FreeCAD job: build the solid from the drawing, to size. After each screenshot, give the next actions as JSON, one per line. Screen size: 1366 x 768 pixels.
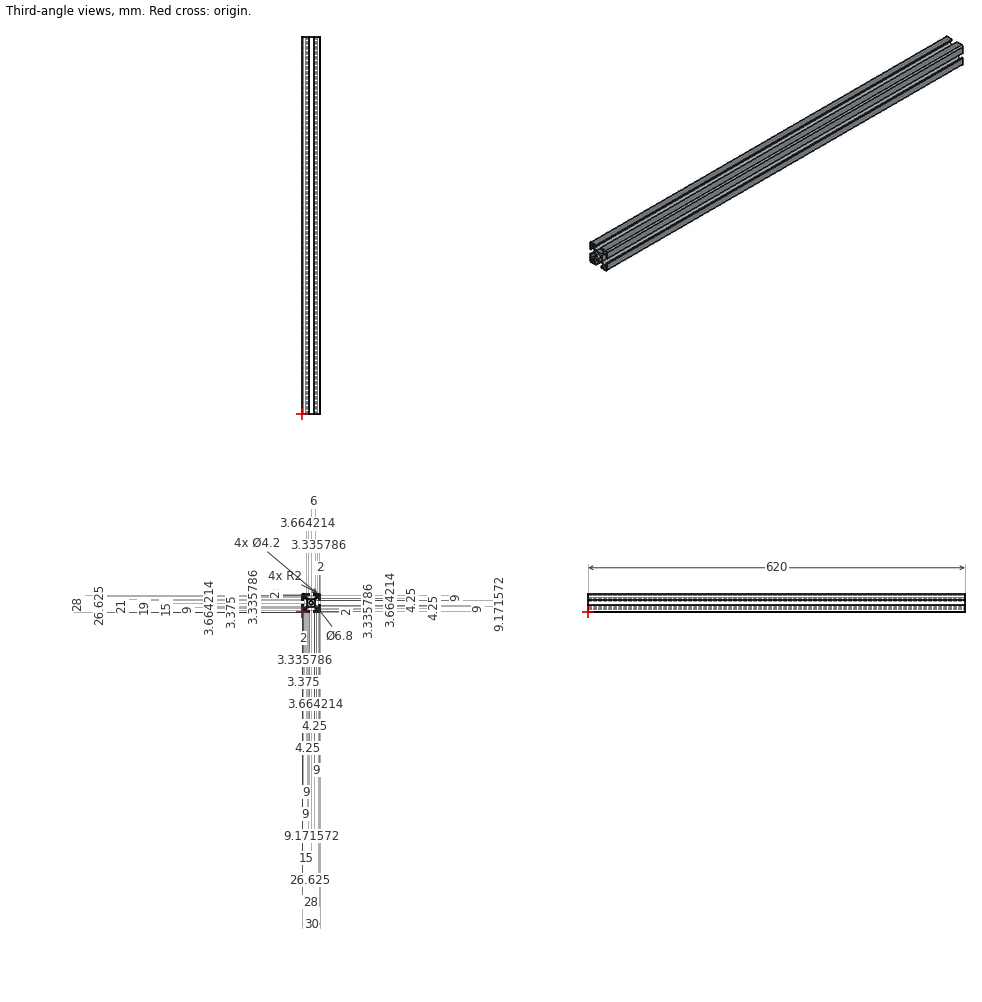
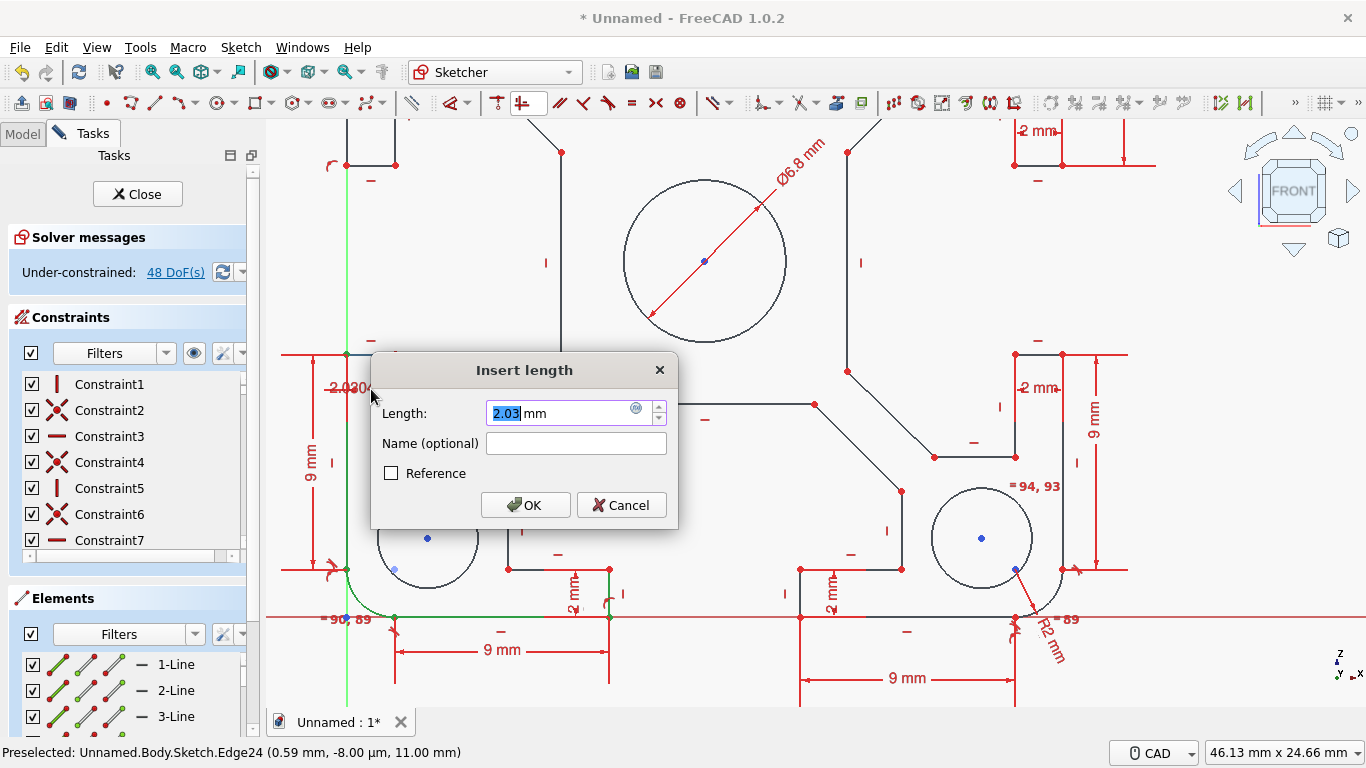
{"action": "type", "text": "2"}
{"action": "key", "text": "Return"}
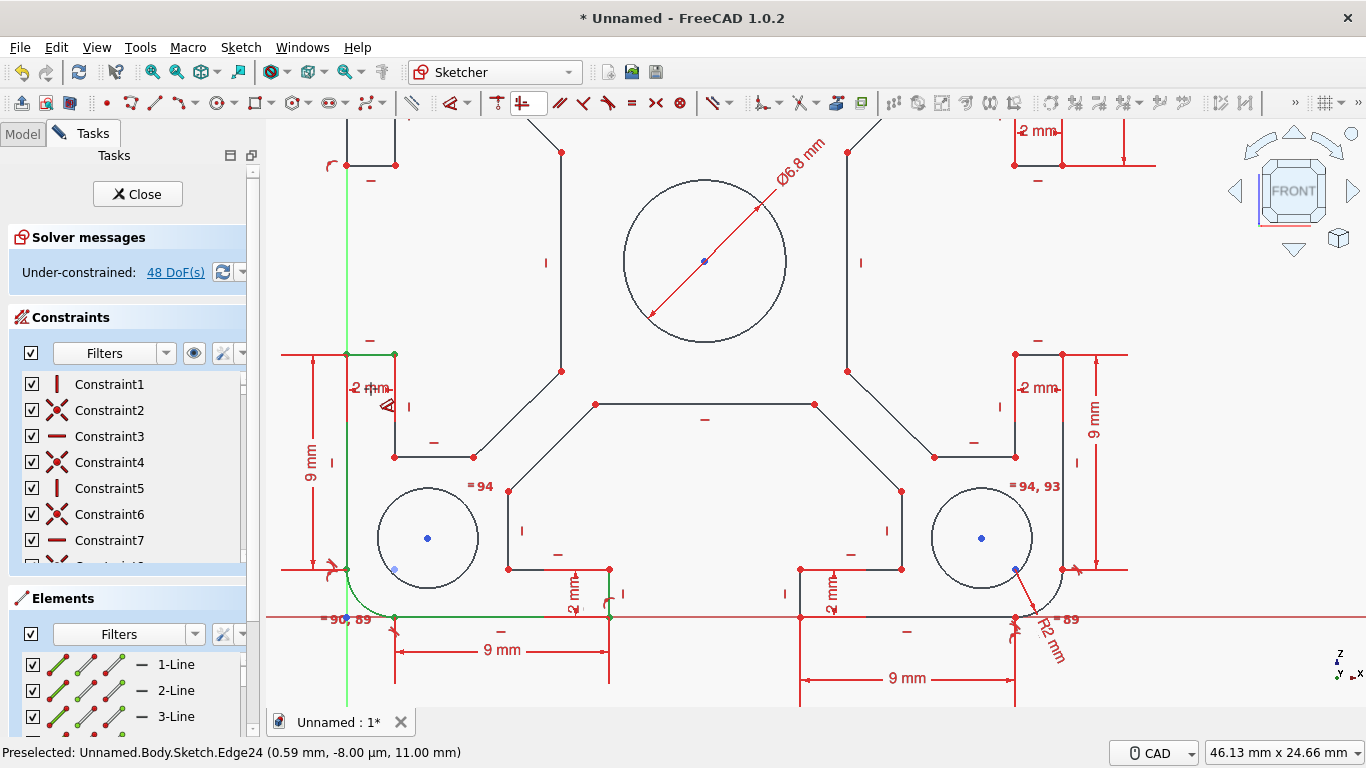
{"action": "left_click", "coordinate": [381, 166]}
{"action": "left_click", "coordinate": [371, 200]}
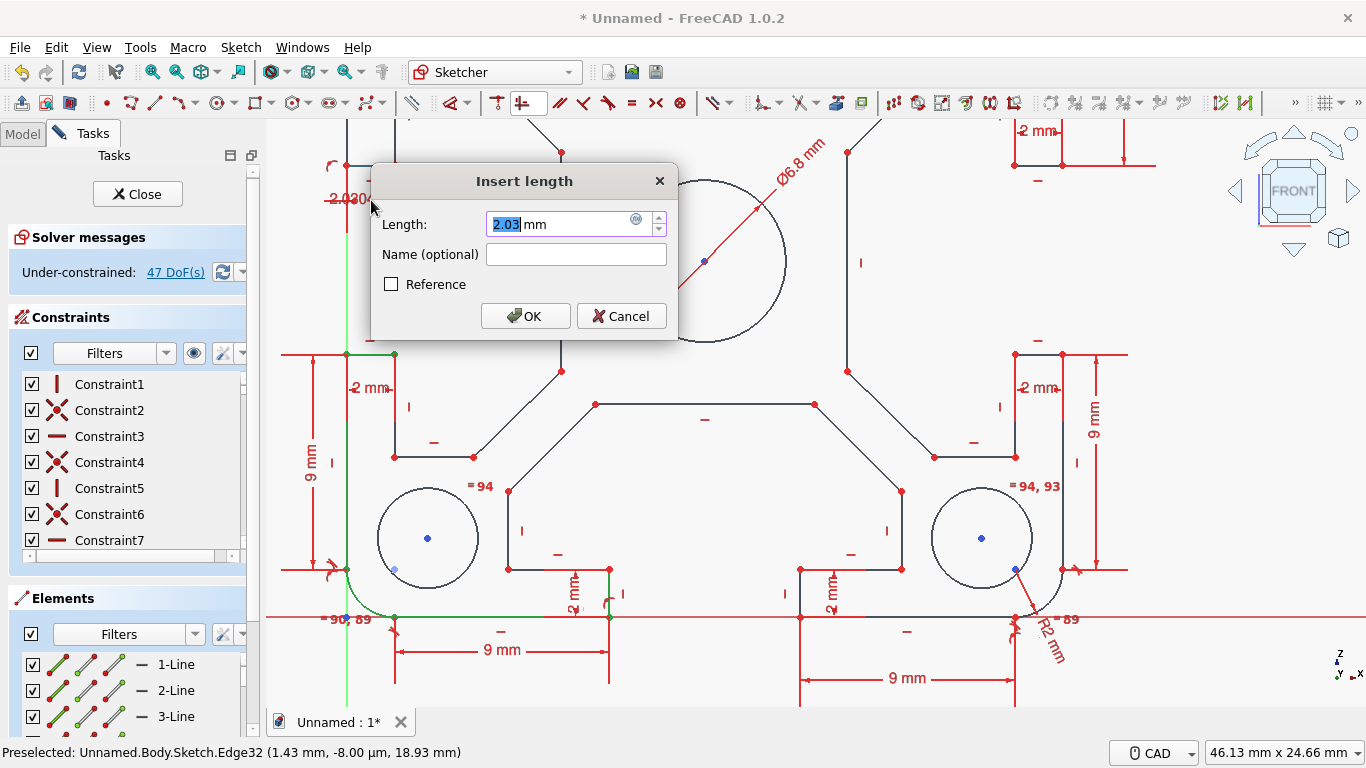
{"action": "type", "text": "2"}
{"action": "key", "text": "Return"}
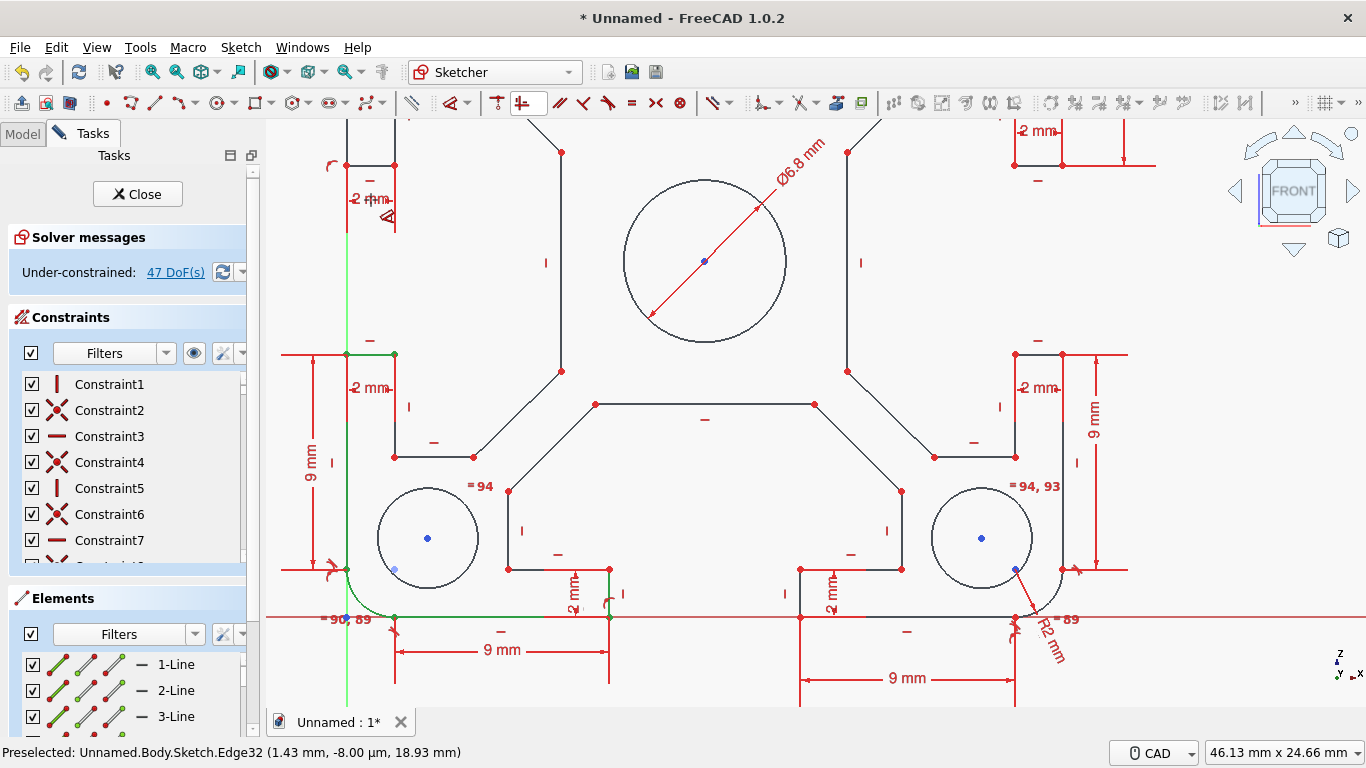
{"action": "scroll", "coordinate": [800, 600], "scroll_direction": "down", "scroll_amount": 3}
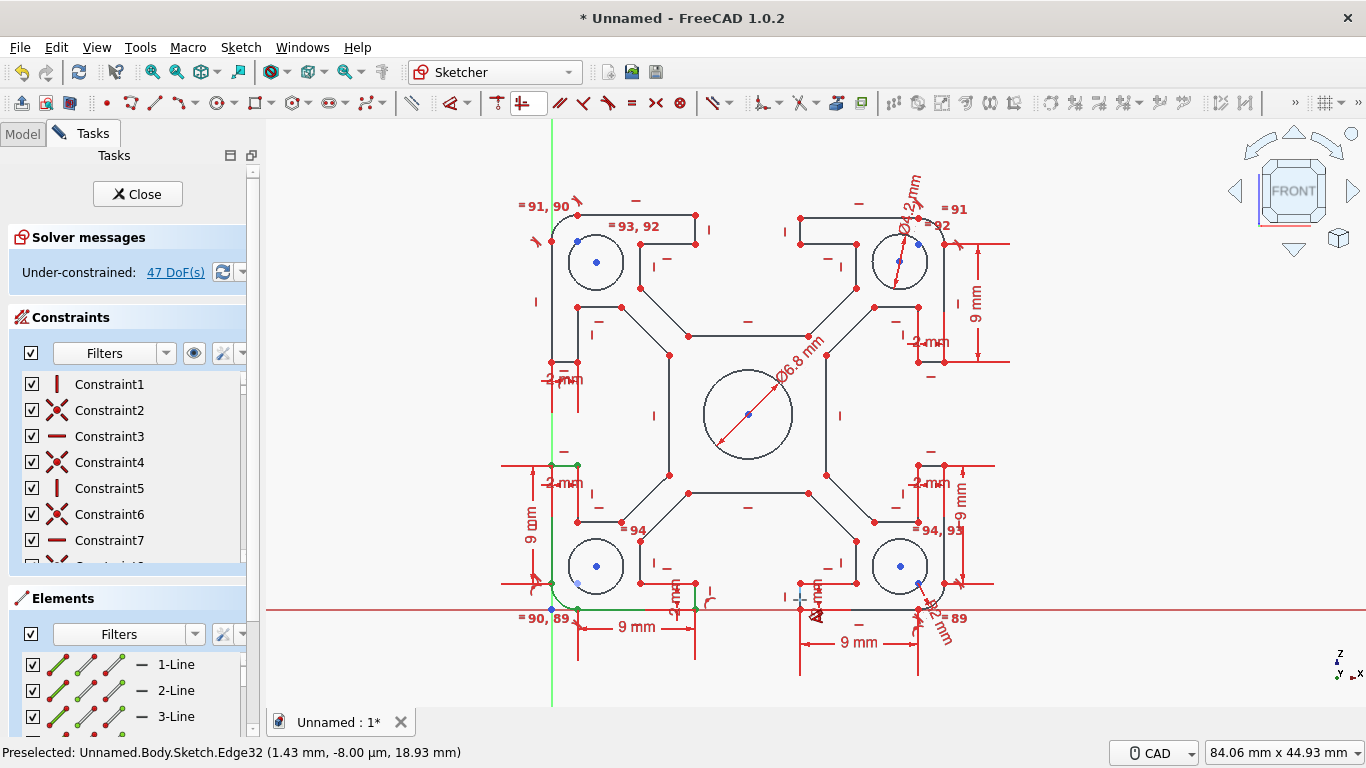
{"action": "left_click", "coordinate": [552, 326]}
{"action": "left_click", "coordinate": [518, 302]}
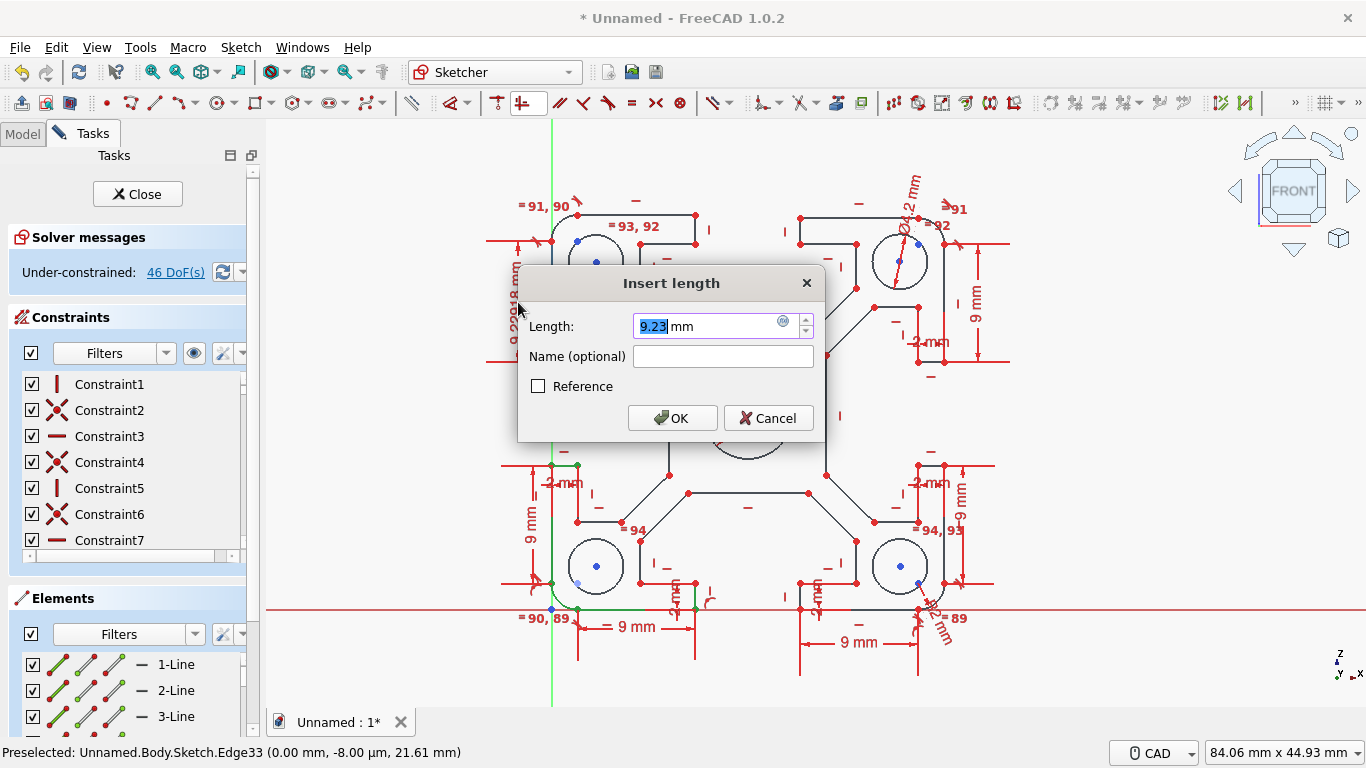
{"action": "type", "text": "9"}
{"action": "key", "text": "Return"}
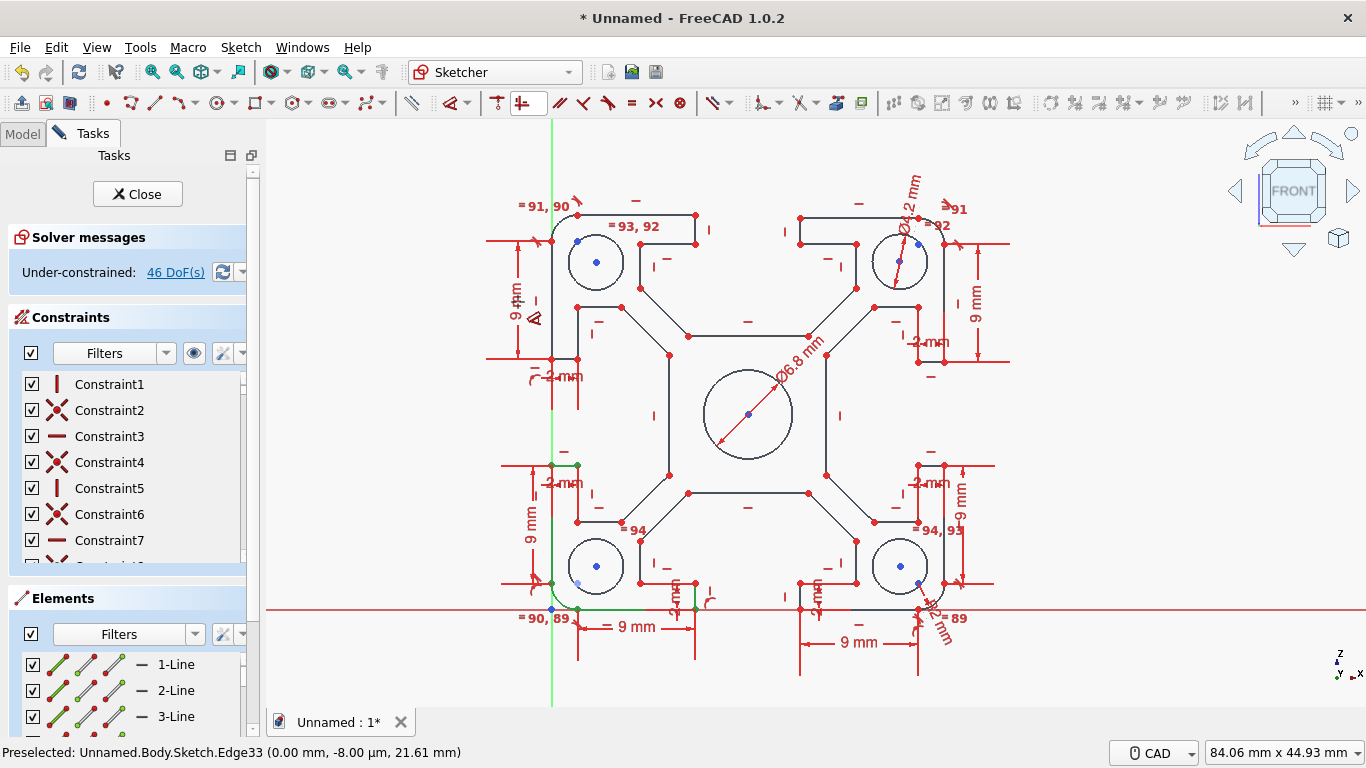
{"action": "left_click", "coordinate": [613, 215]}
{"action": "left_click", "coordinate": [636, 181]}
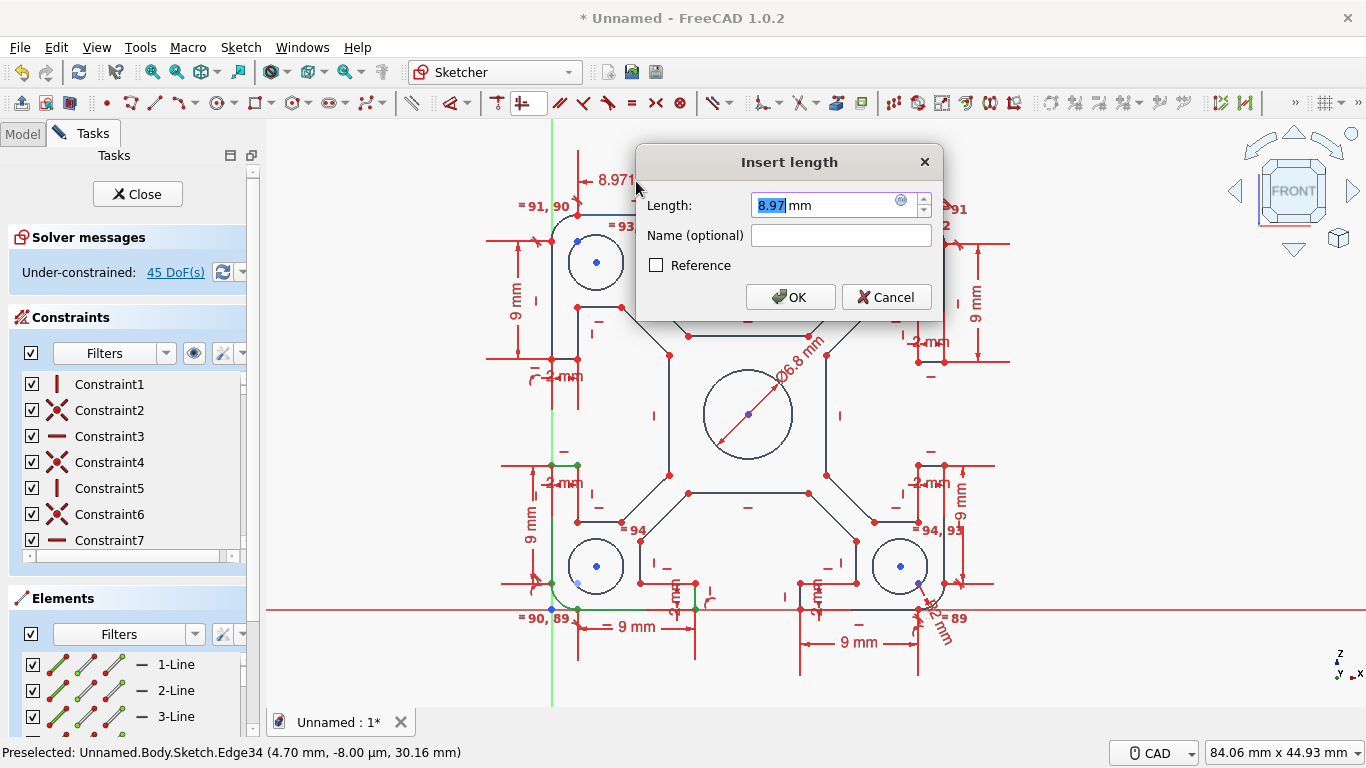
{"action": "type", "text": "9"}
{"action": "key", "text": "Return"}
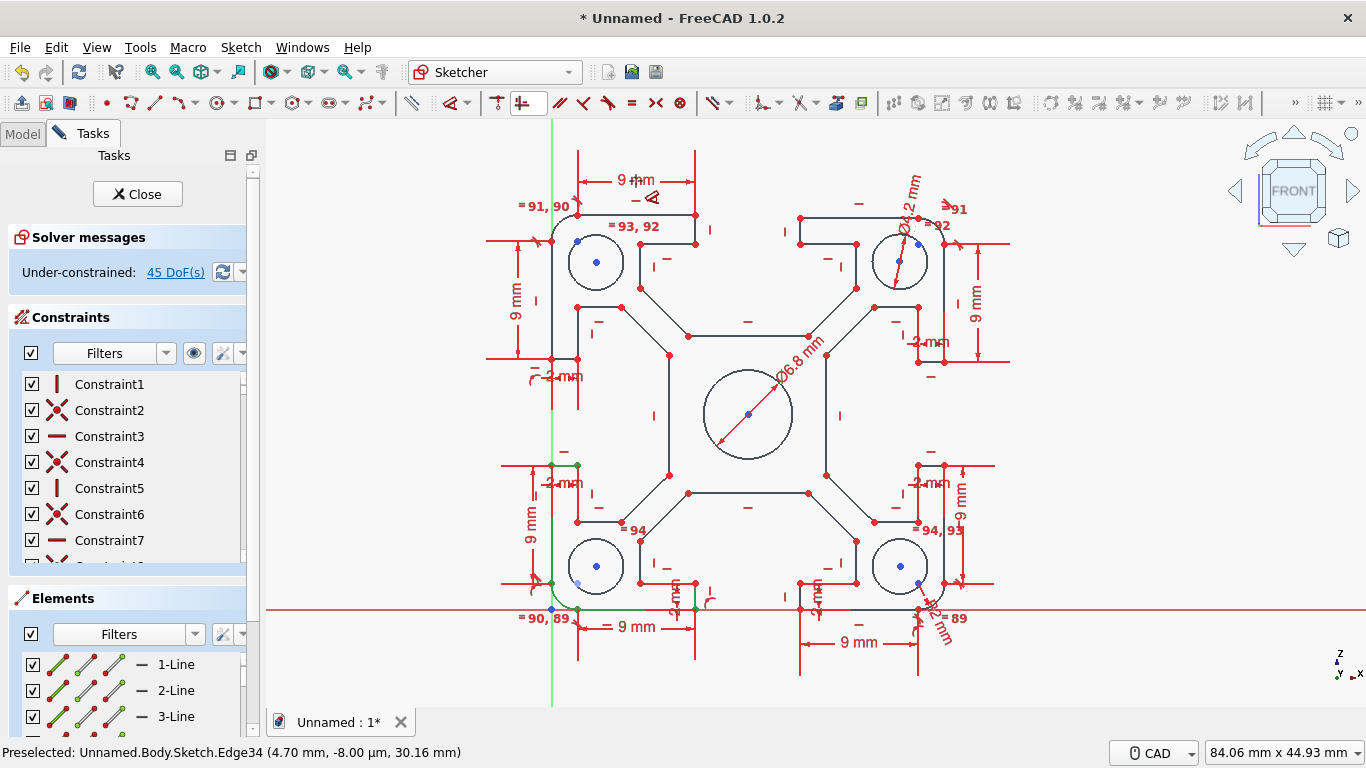
{"action": "scroll", "coordinate": [695, 227], "scroll_direction": "up", "scroll_amount": 3}